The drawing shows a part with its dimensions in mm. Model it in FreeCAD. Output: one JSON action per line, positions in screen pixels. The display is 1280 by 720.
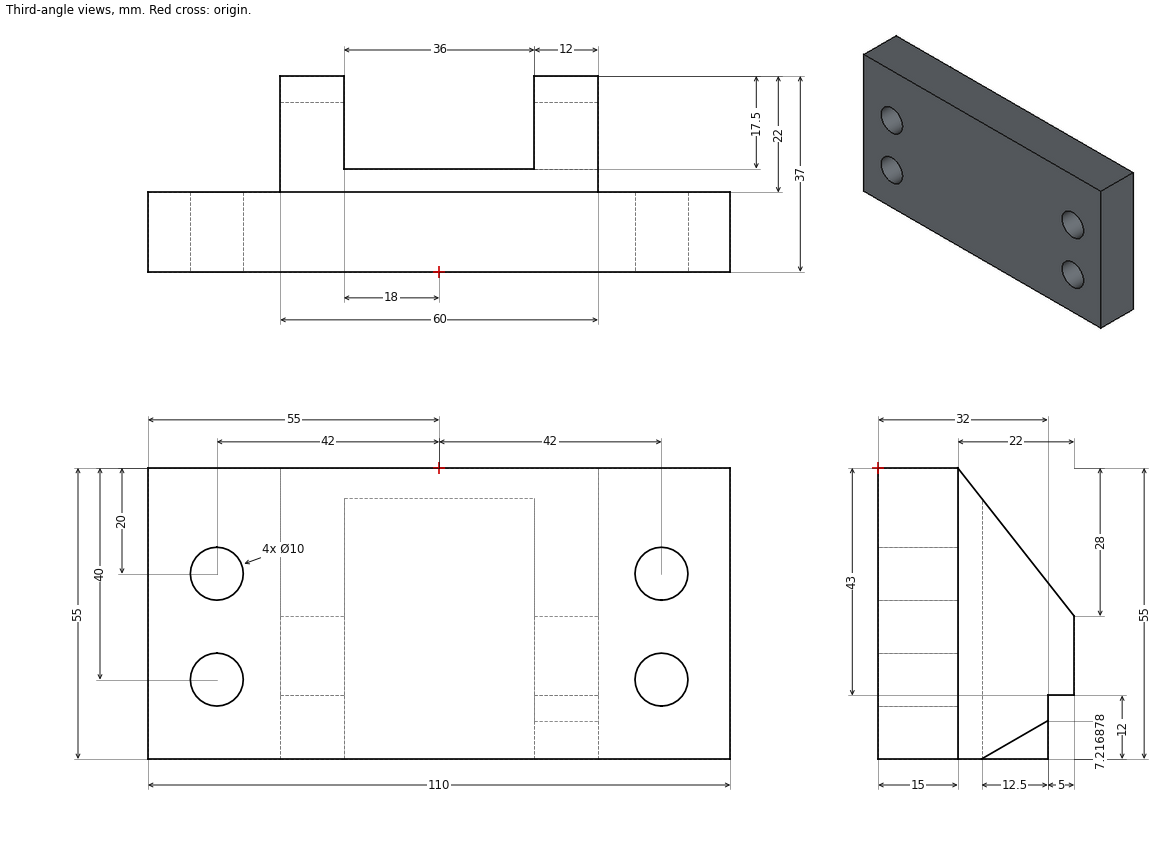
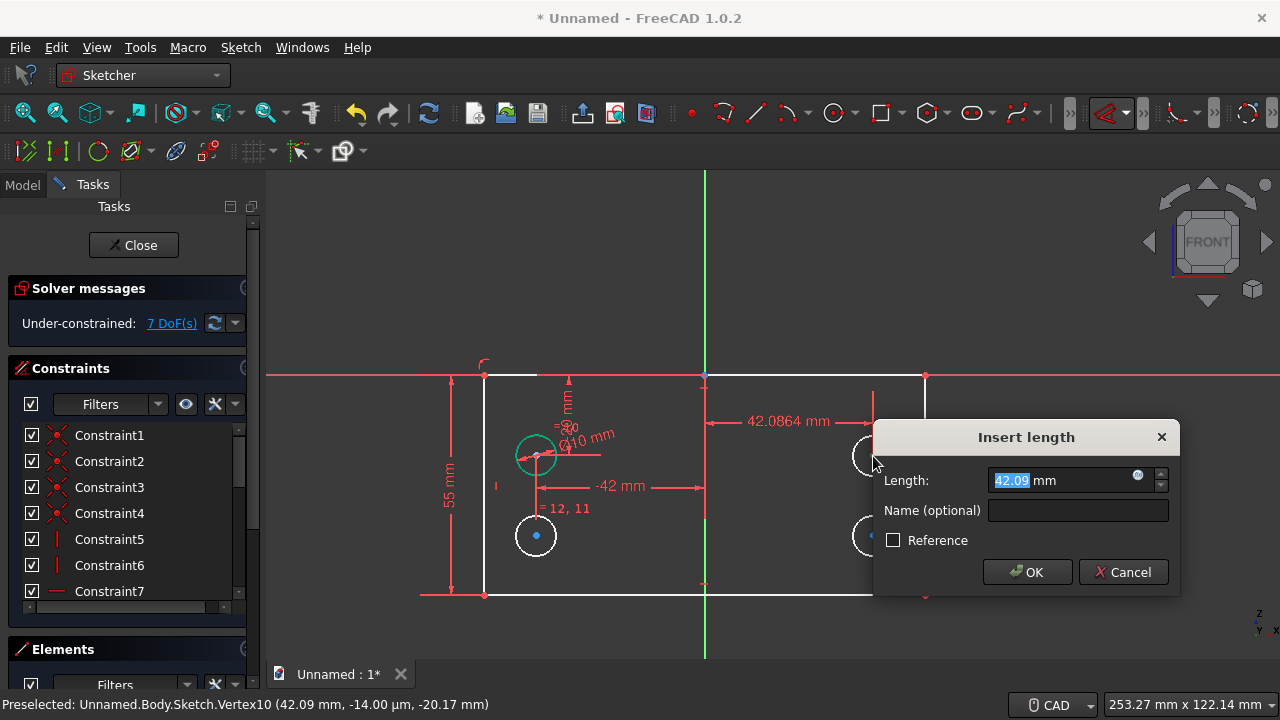
{"action": "type", "text": "42"}
{"action": "key", "text": "Return"}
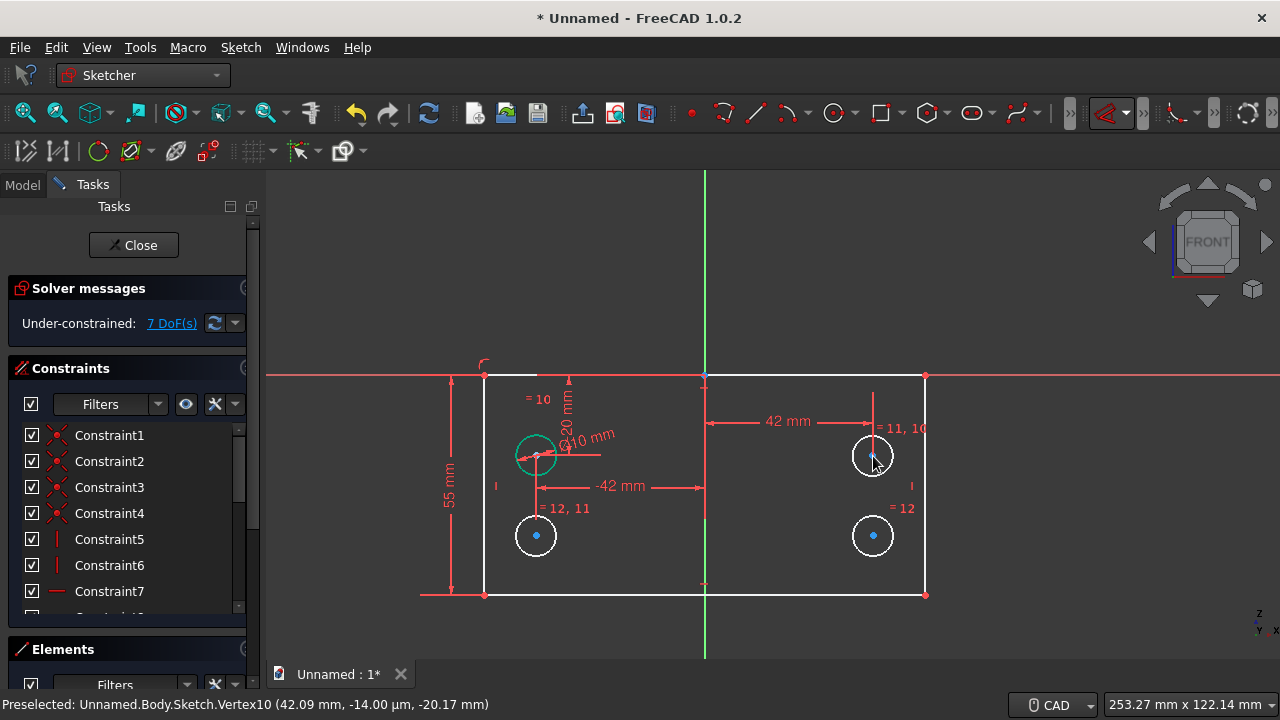
{"action": "left_click", "coordinate": [873, 456]}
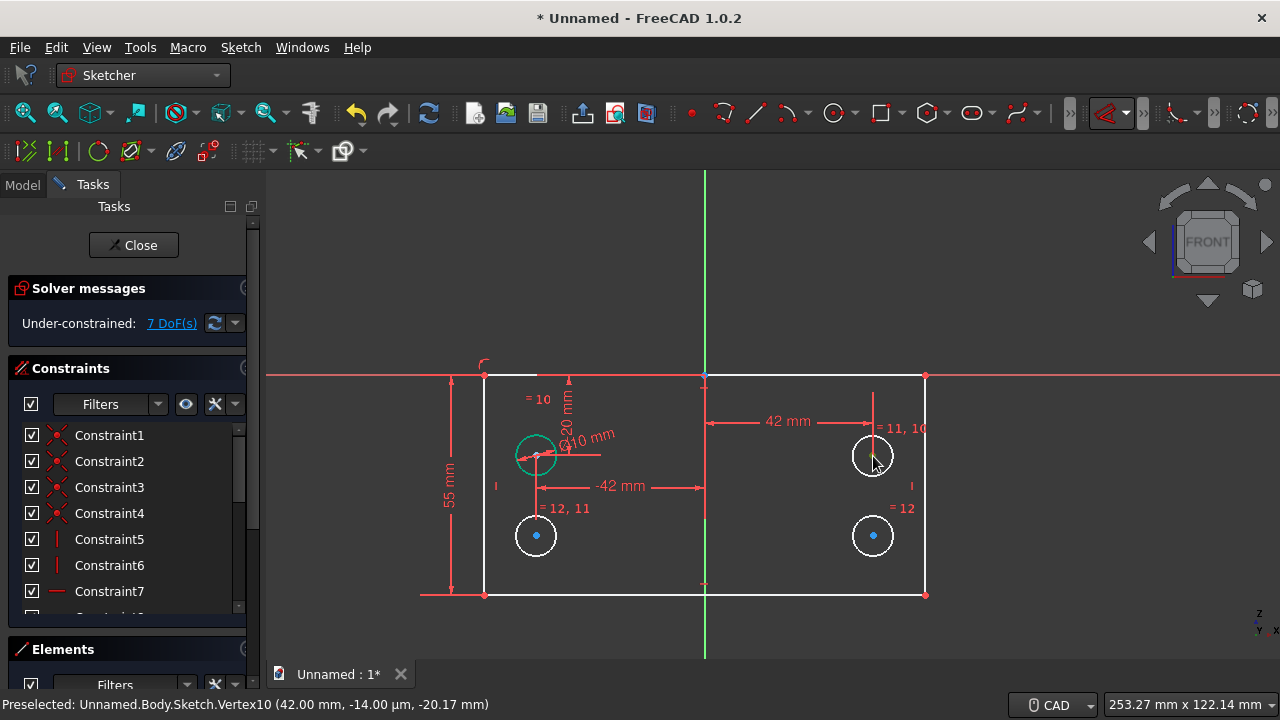
{"action": "left_click", "coordinate": [1128, 114]}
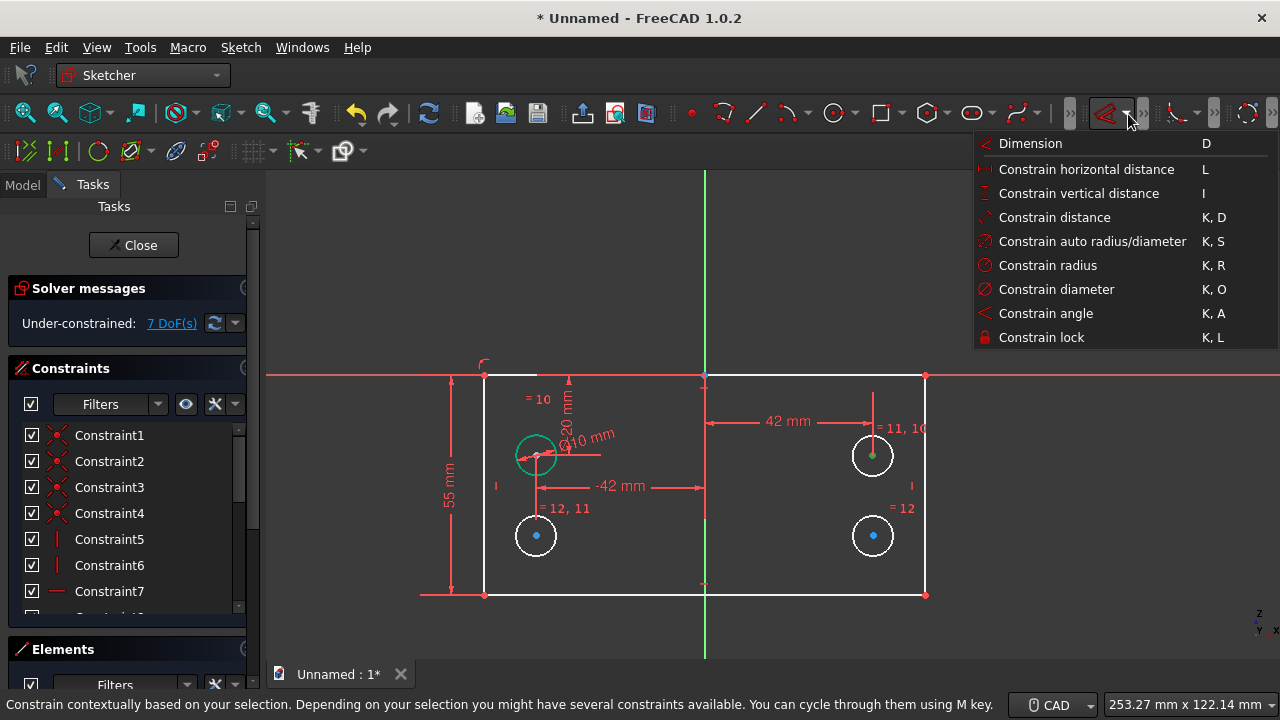
{"action": "left_click", "coordinate": [1126, 193]}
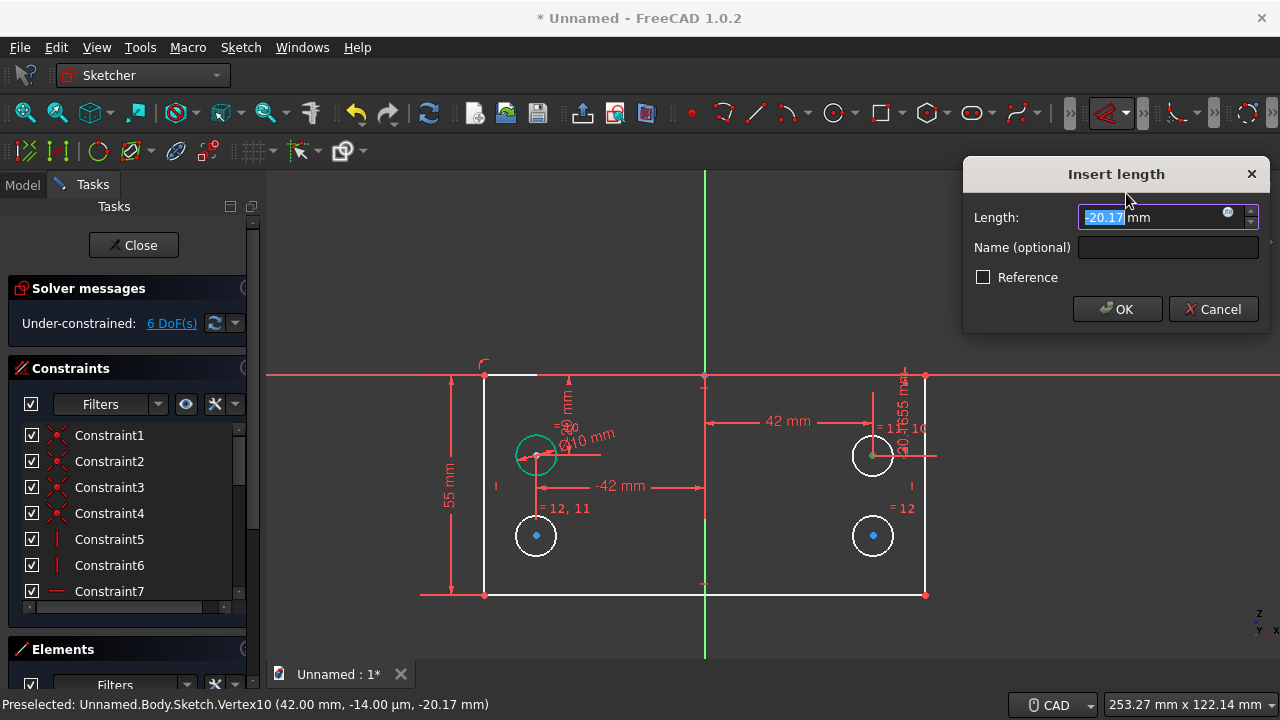
{"action": "type", "text": "-20"}
{"action": "key", "text": "Return"}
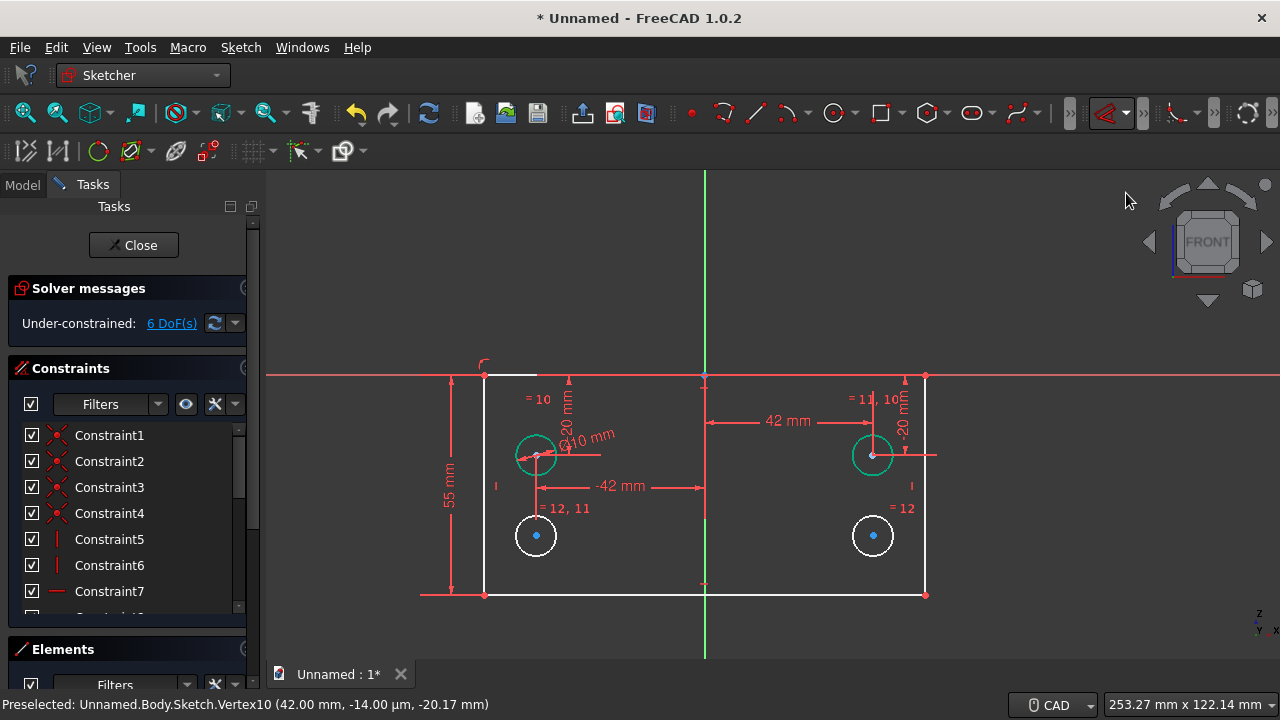
{"action": "left_click", "coordinate": [536, 536]}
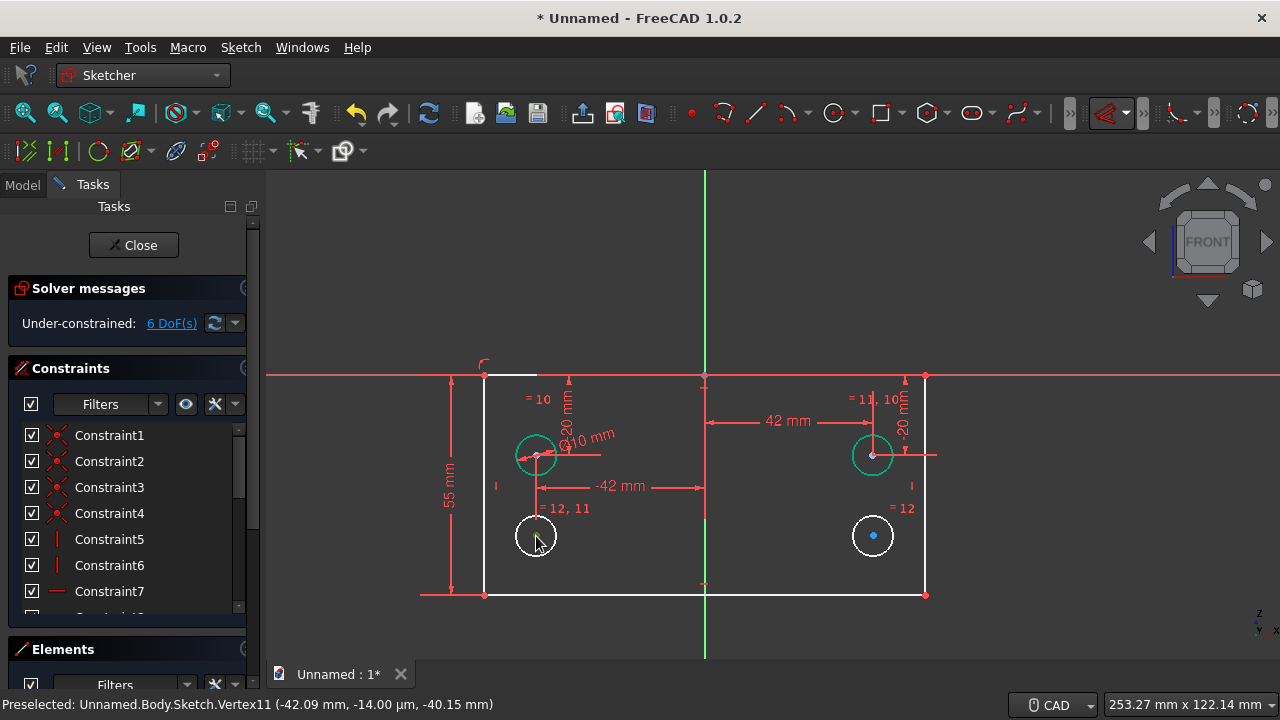
{"action": "left_click", "coordinate": [1128, 114]}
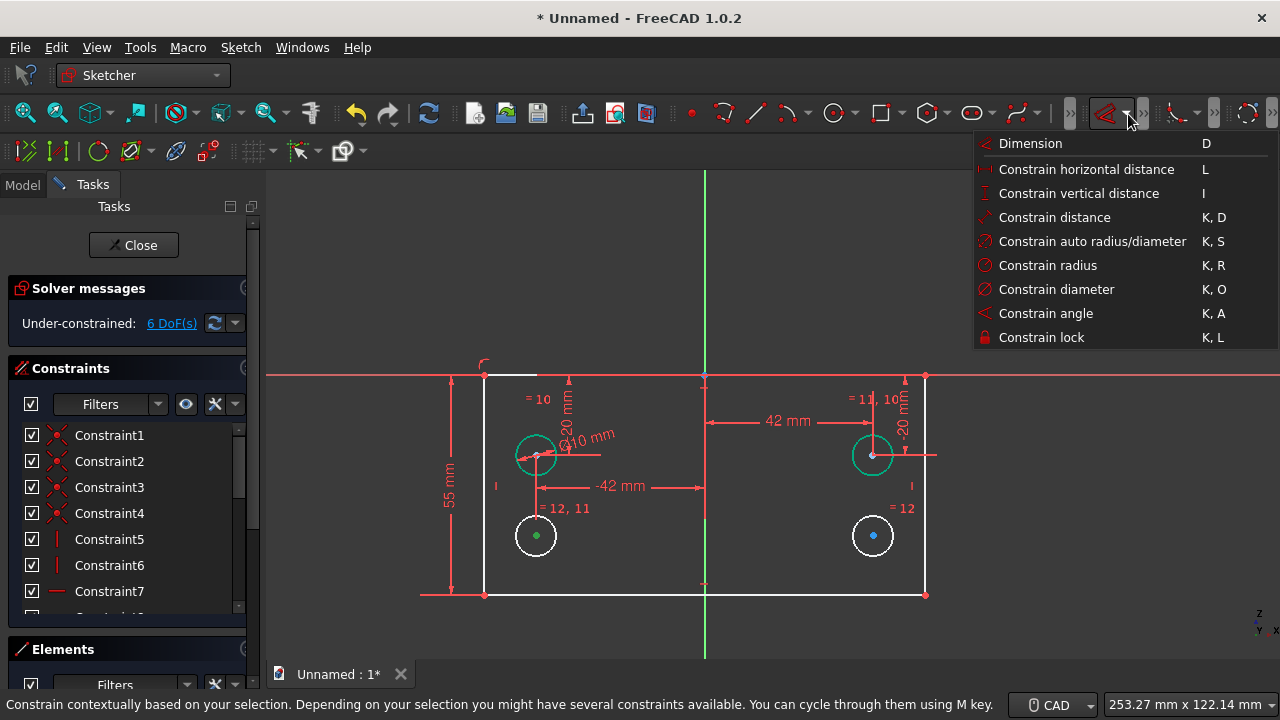
{"action": "left_click", "coordinate": [1126, 169]}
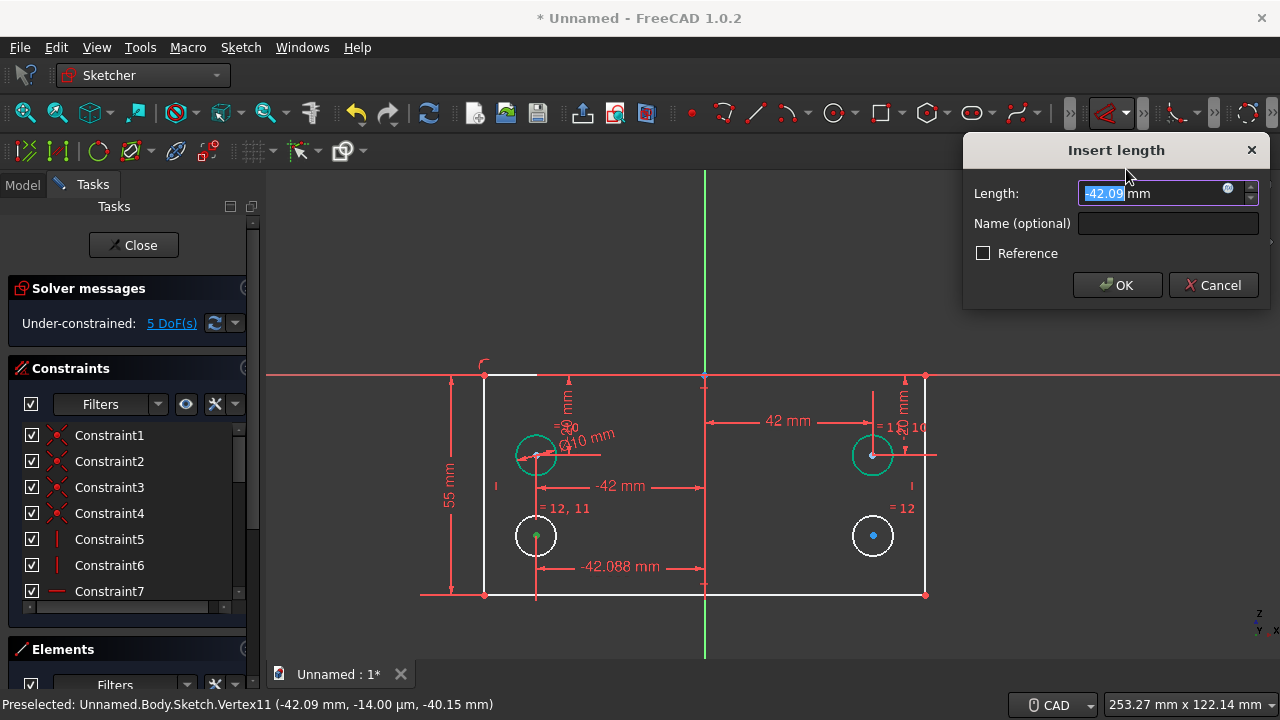
{"action": "type", "text": "-42"}
{"action": "key", "text": "Return"}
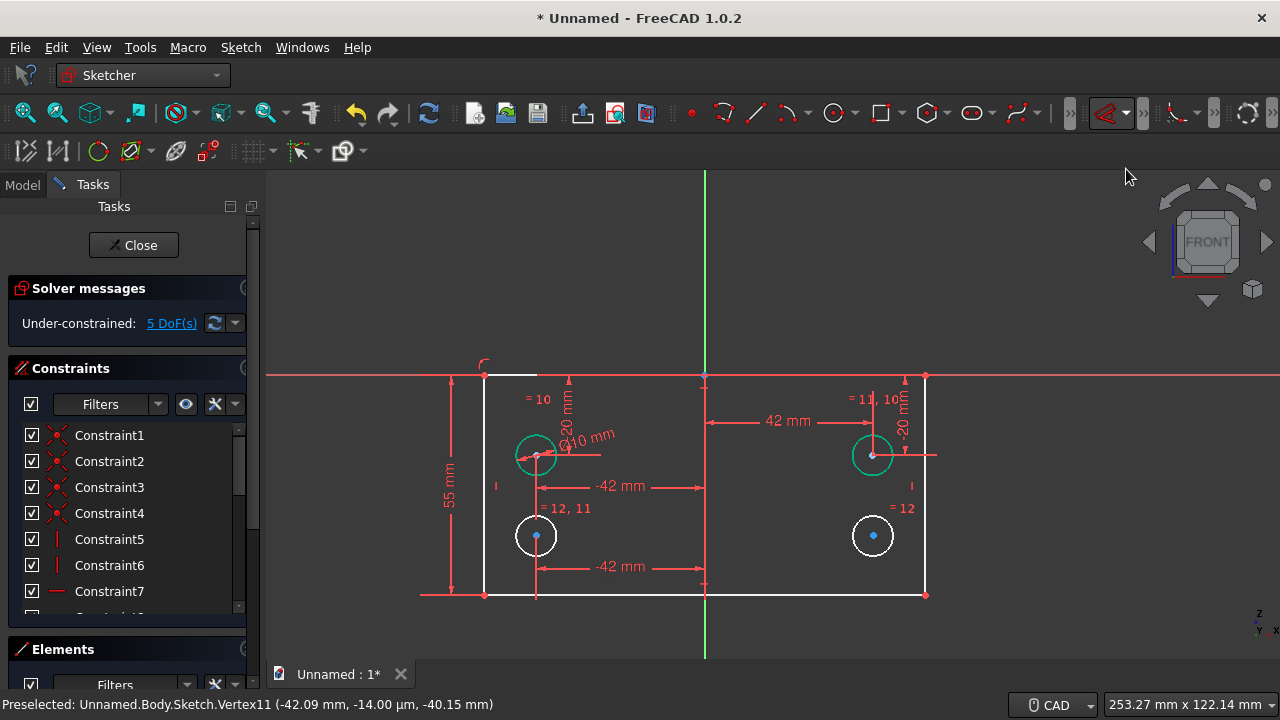
{"action": "left_click", "coordinate": [536, 536]}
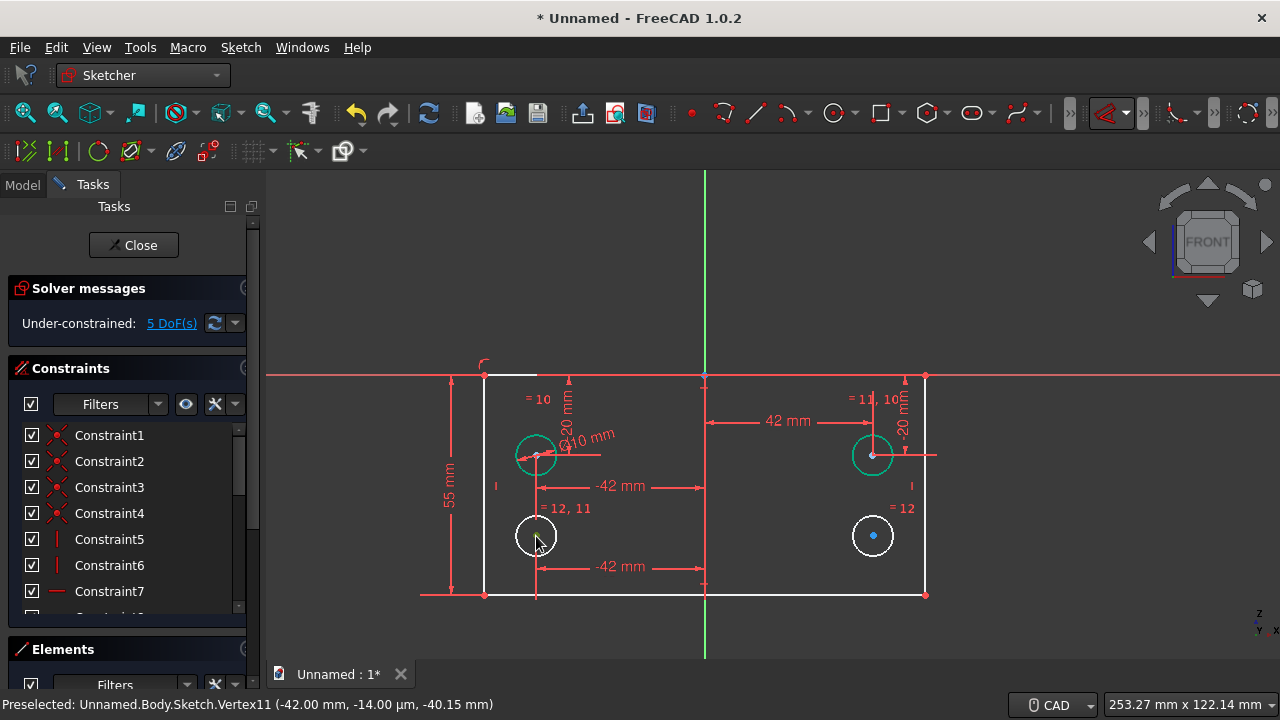
{"action": "left_click", "coordinate": [1128, 114]}